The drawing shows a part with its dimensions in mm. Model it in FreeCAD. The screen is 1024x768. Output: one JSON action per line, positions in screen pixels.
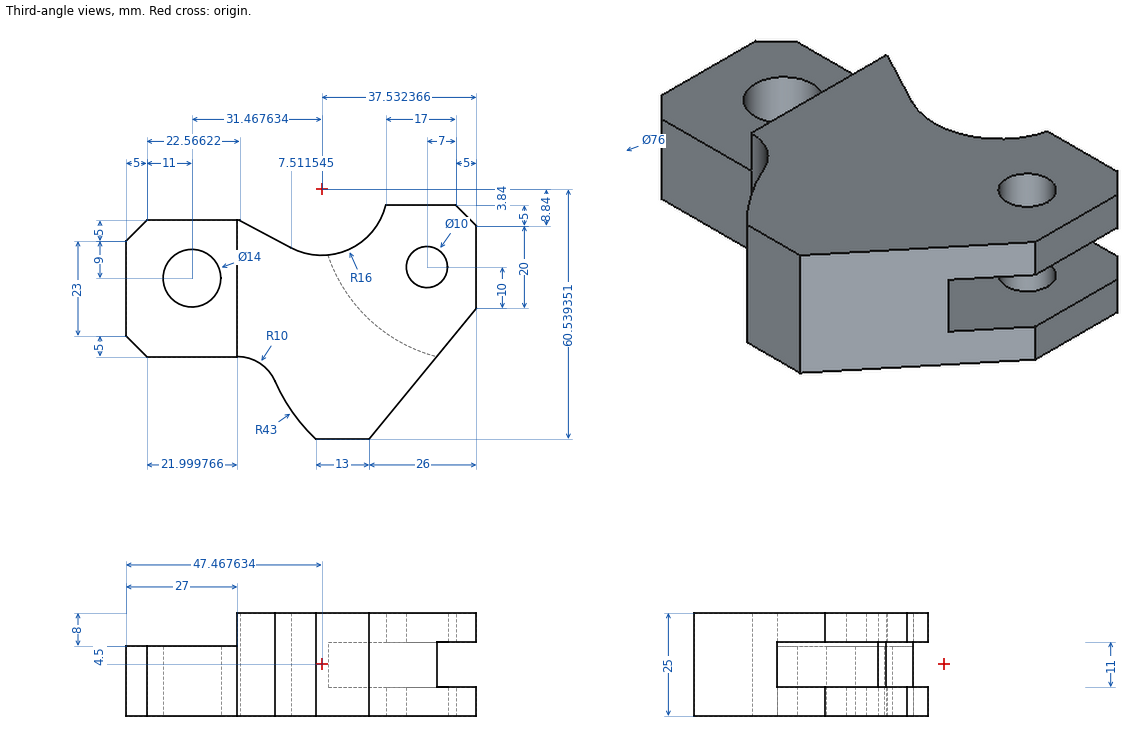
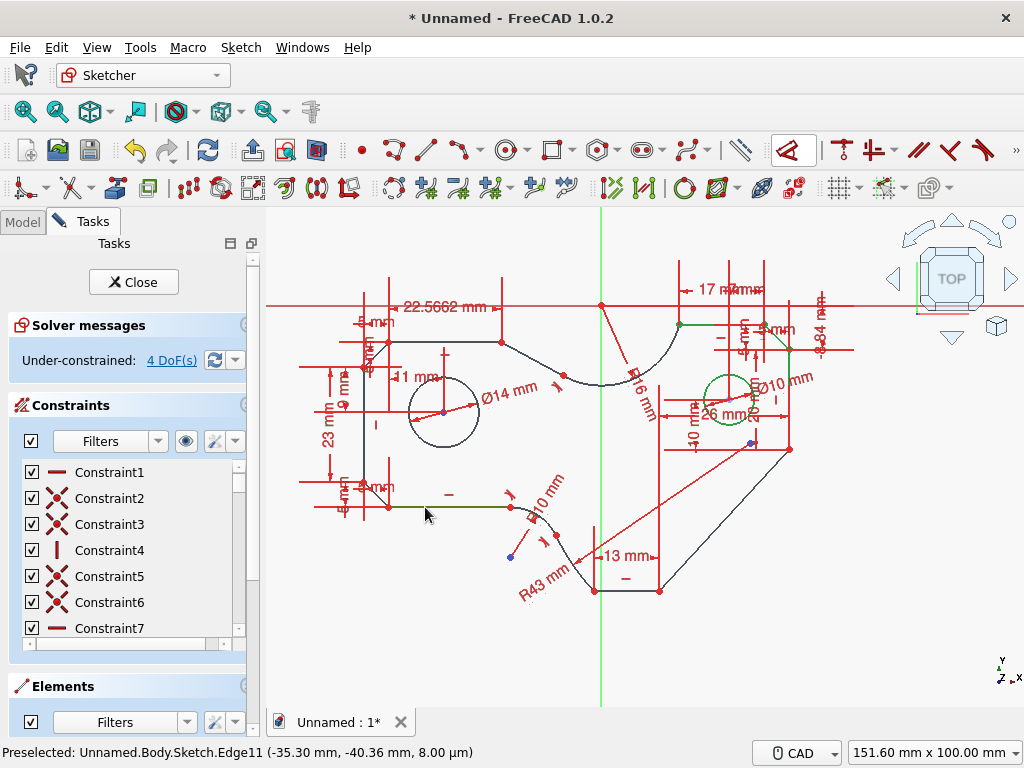
{"action": "key", "text": "l"}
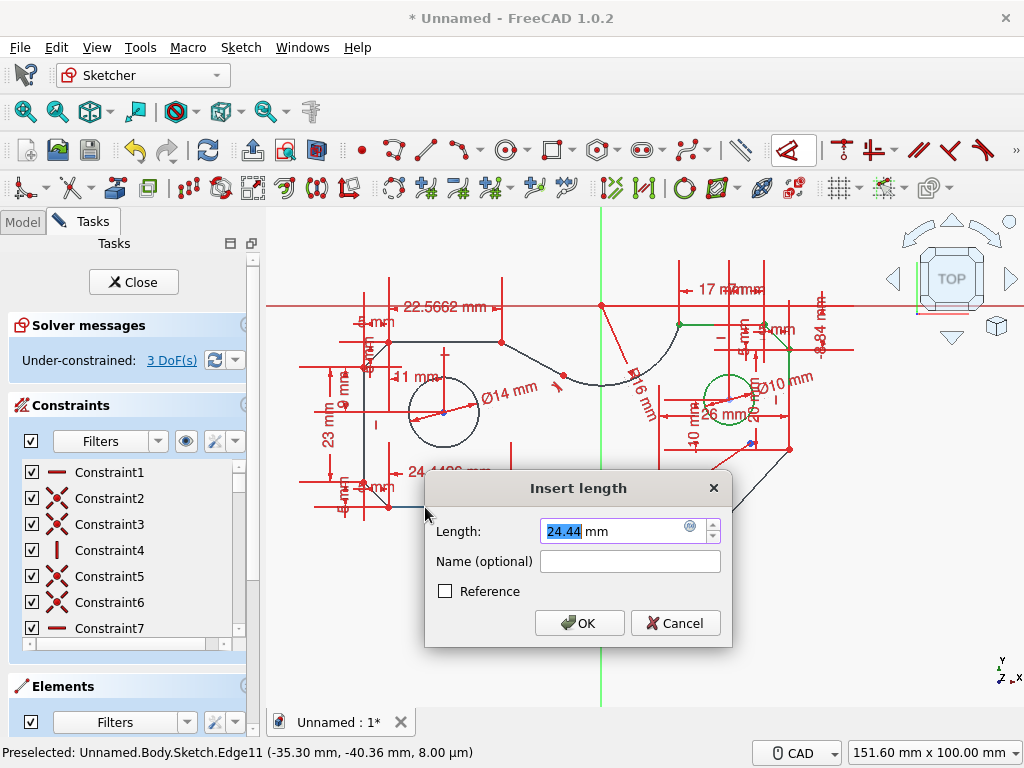
{"action": "type", "text": "21.999766"}
{"action": "key", "text": "Return"}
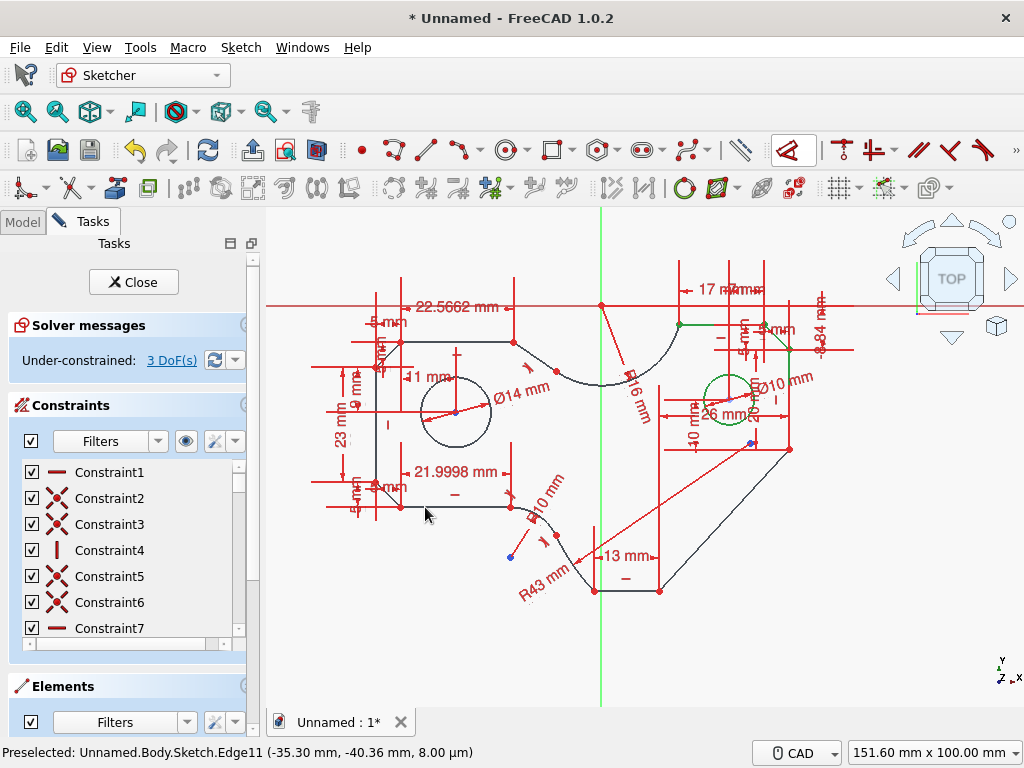
{"action": "left_click", "coordinate": [556, 372]}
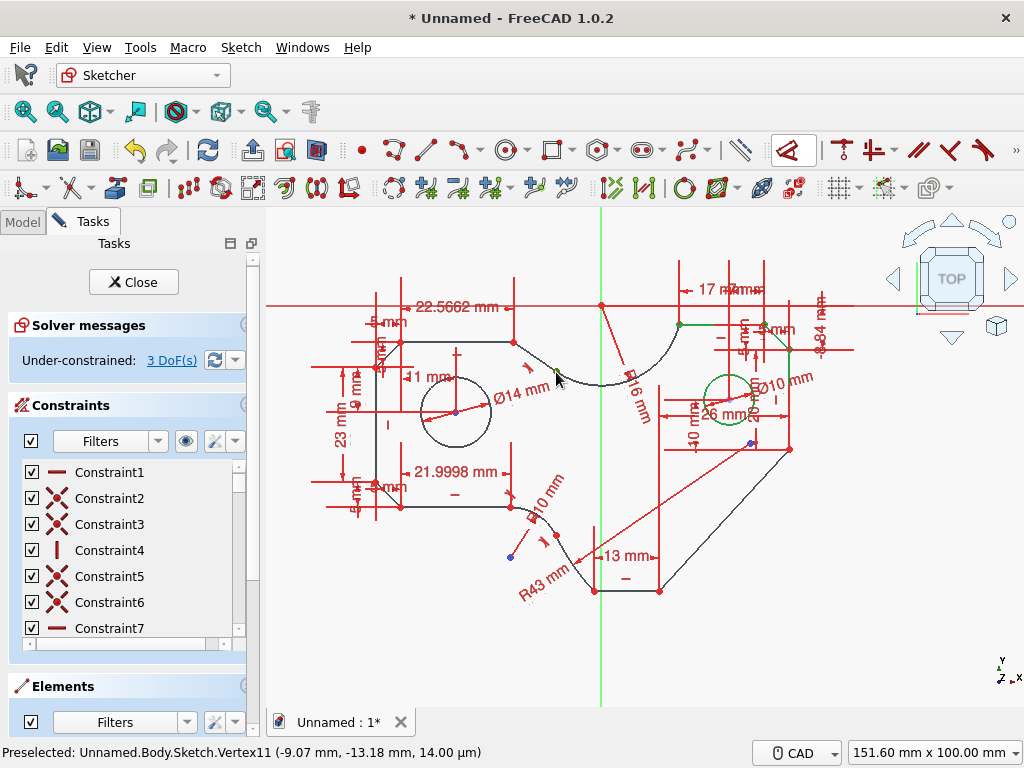
{"action": "key", "text": "l"}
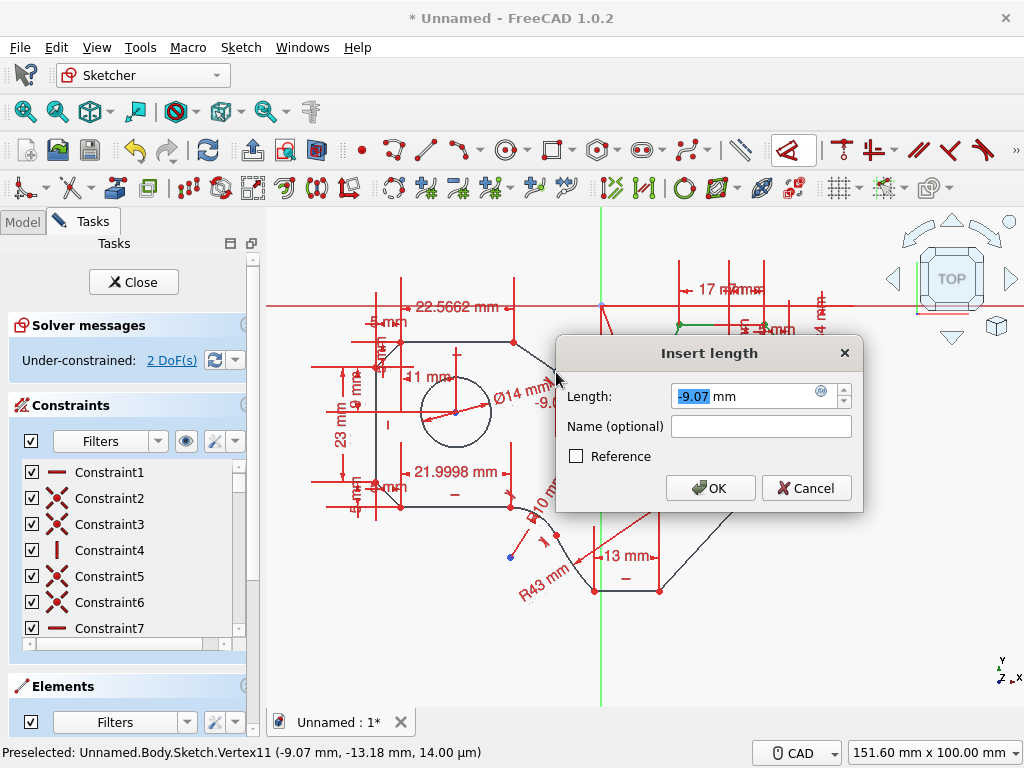
{"action": "type", "text": "-7.511545"}
{"action": "key", "text": "Return"}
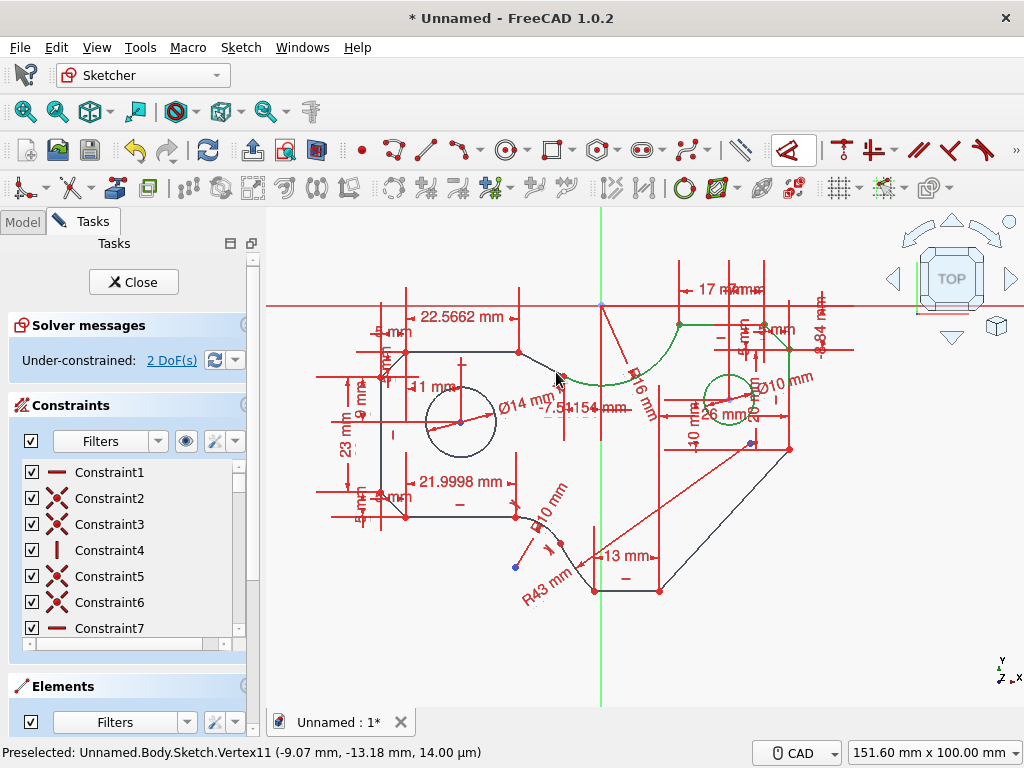
{"action": "left_click", "coordinate": [461, 422]}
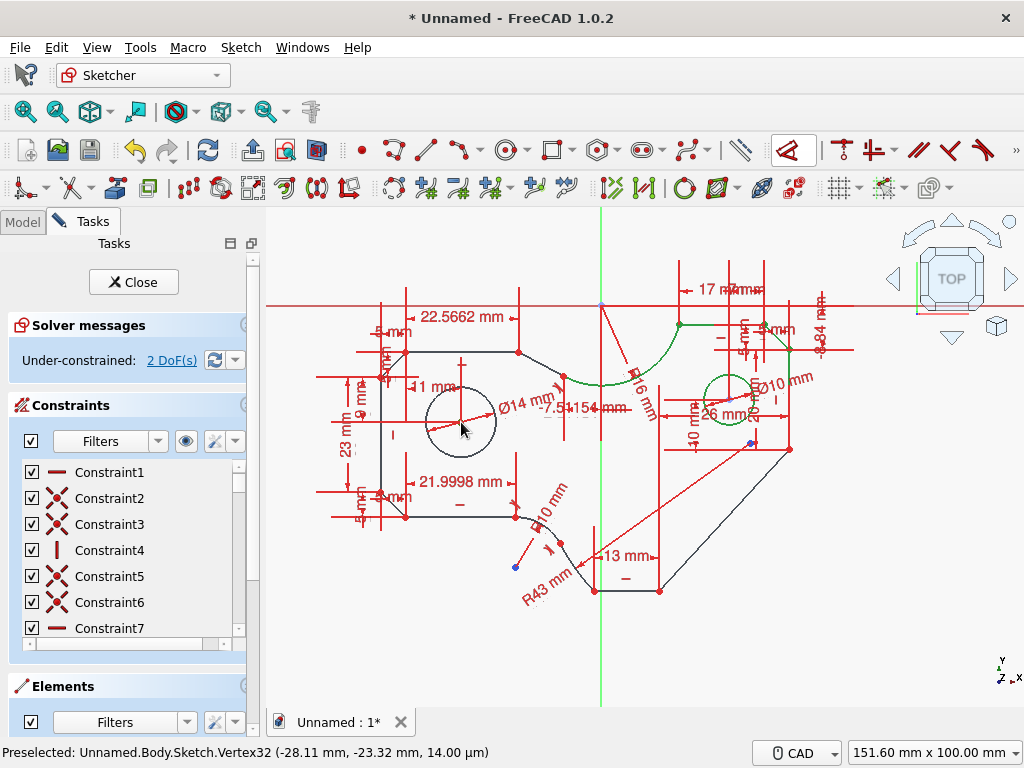
{"action": "left_click", "coordinate": [810, 150]}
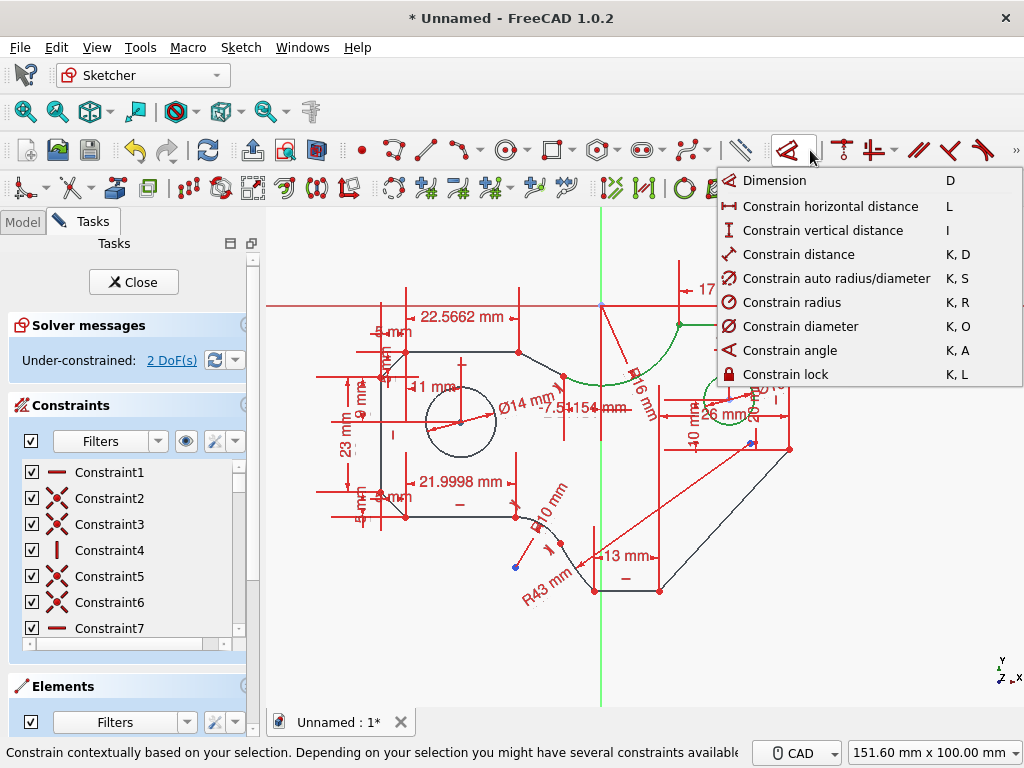
{"action": "left_click", "coordinate": [870, 206]}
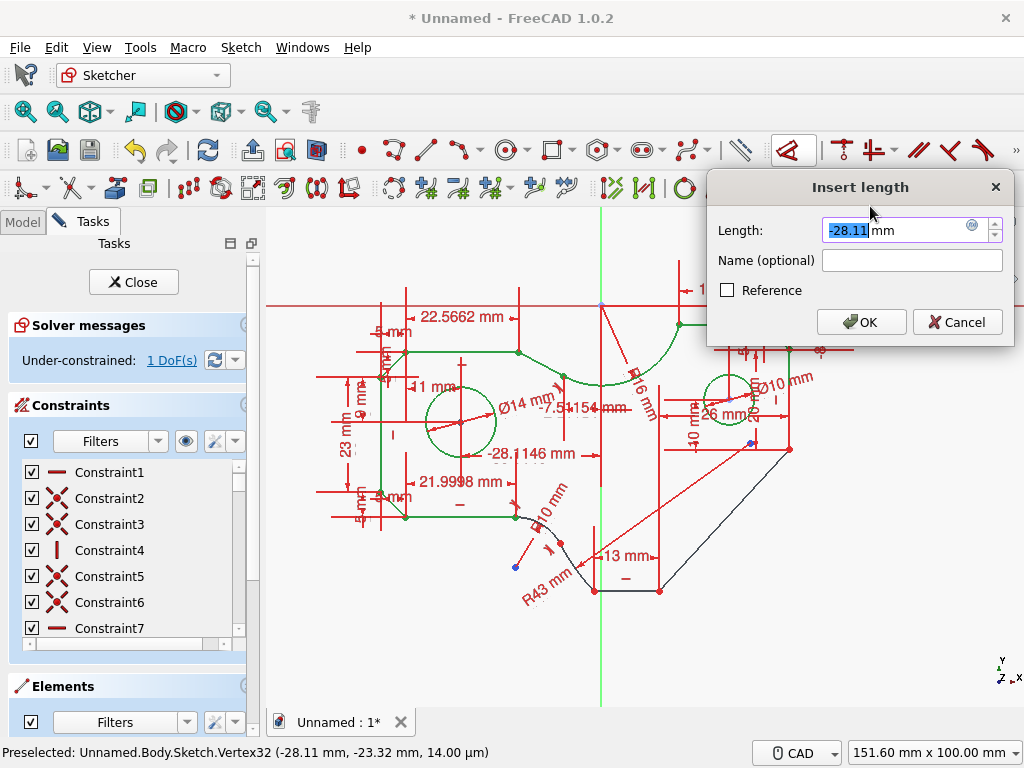
{"action": "type", "text": "-31.467634"}
{"action": "key", "text": "Return"}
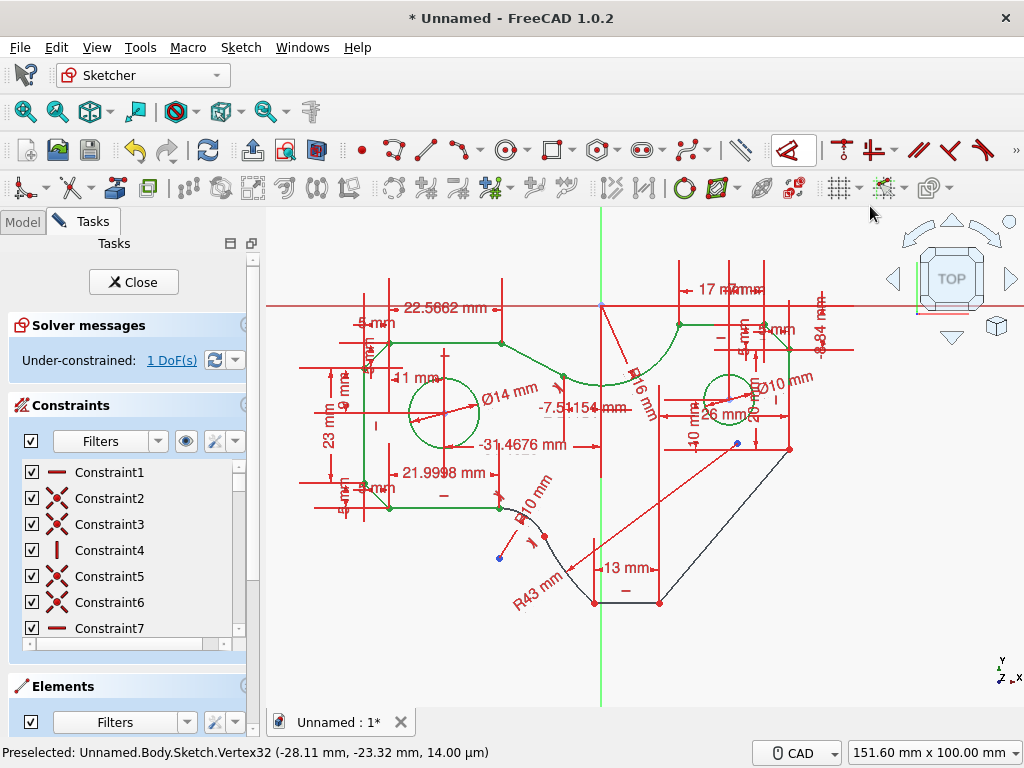
{"action": "left_click", "coordinate": [594, 603]}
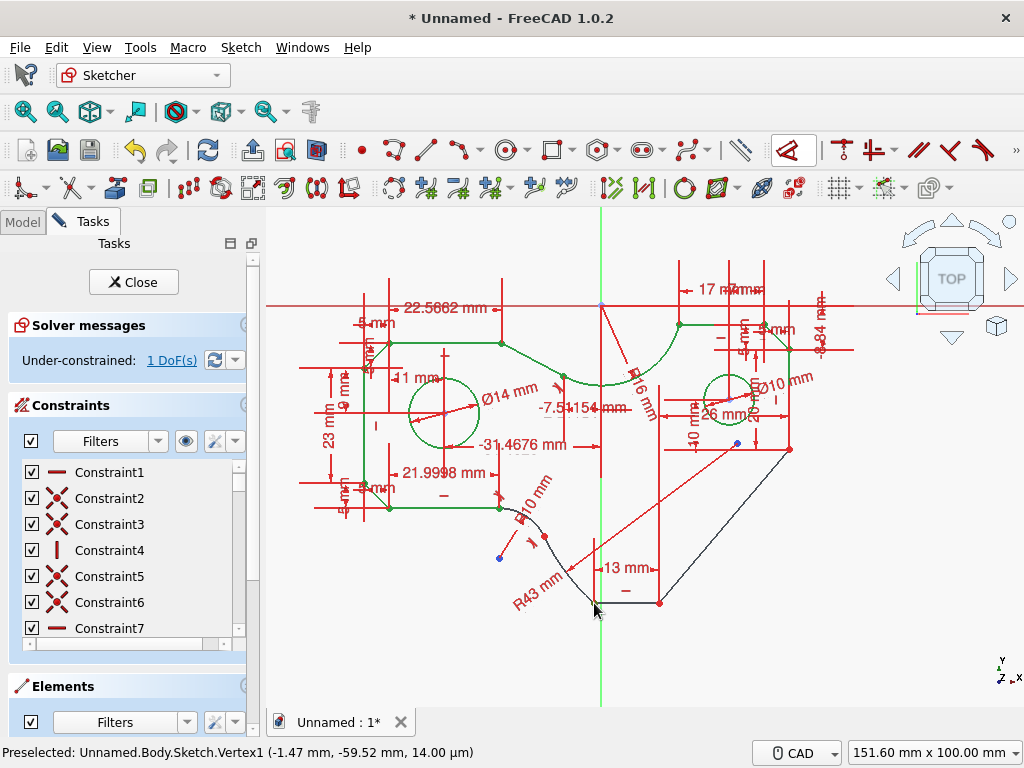
{"action": "key", "text": "i"}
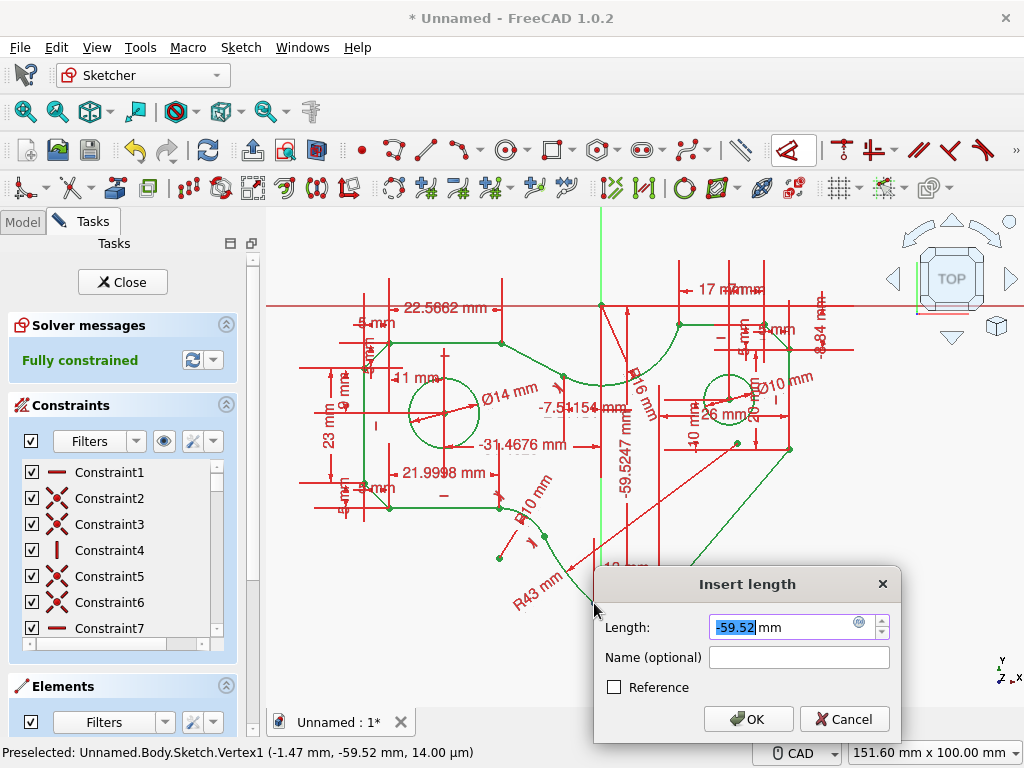
{"action": "type", "text": "-60.539351"}
{"action": "key", "text": "Return"}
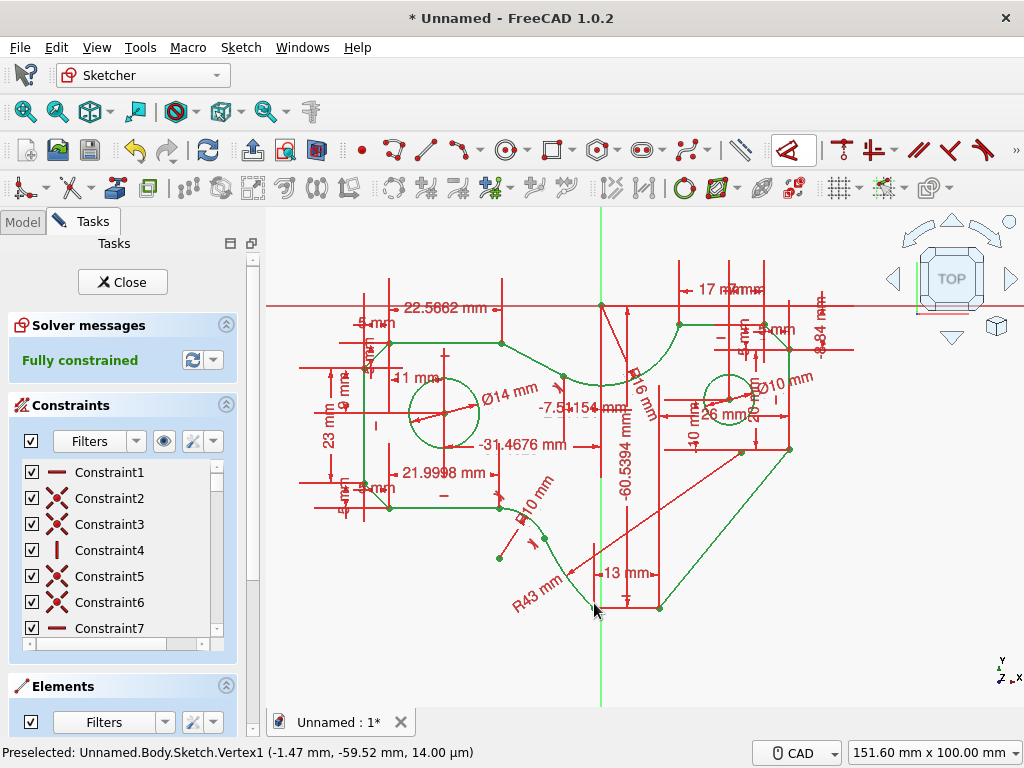
{"action": "left_click", "coordinate": [123, 282]}